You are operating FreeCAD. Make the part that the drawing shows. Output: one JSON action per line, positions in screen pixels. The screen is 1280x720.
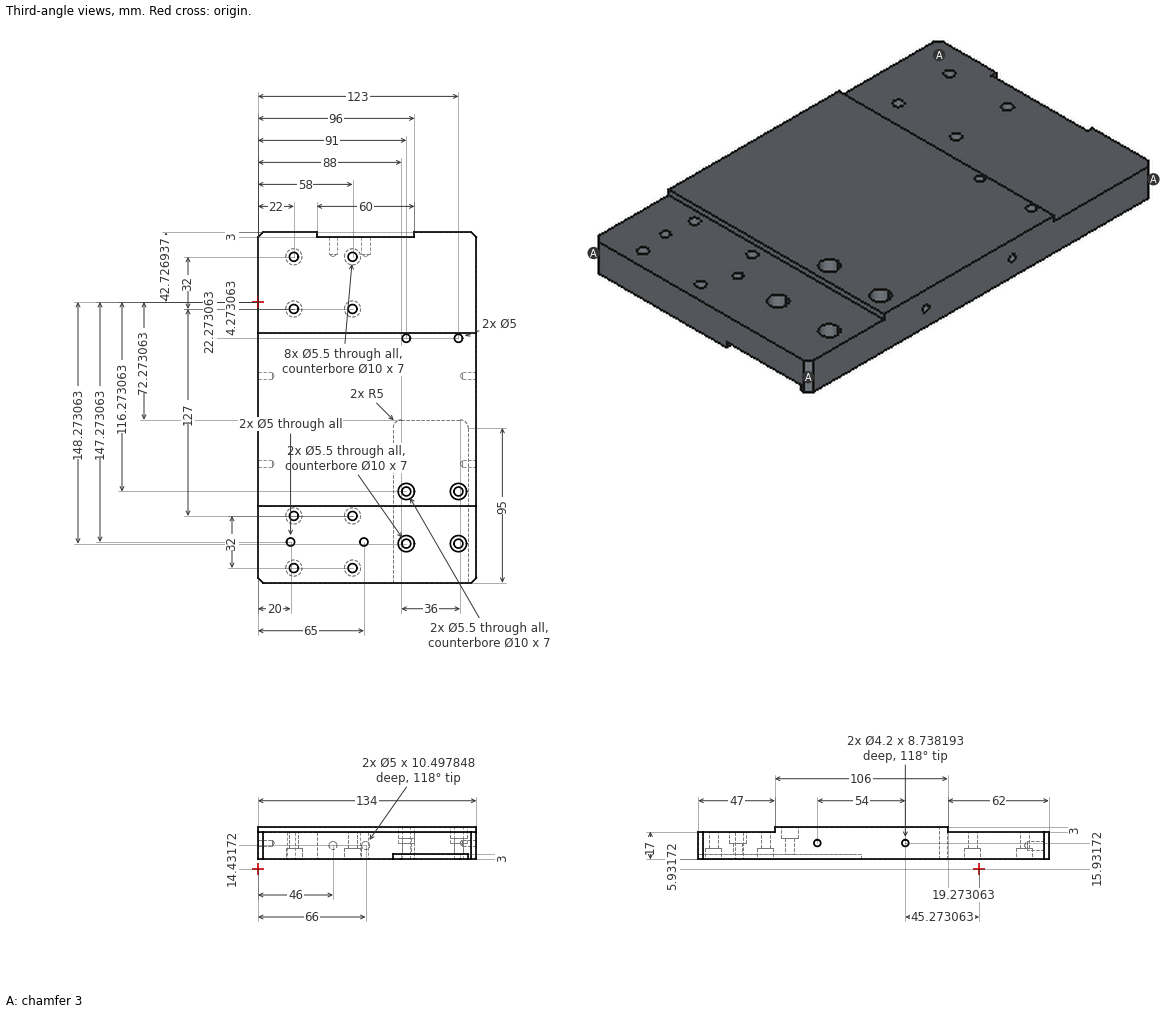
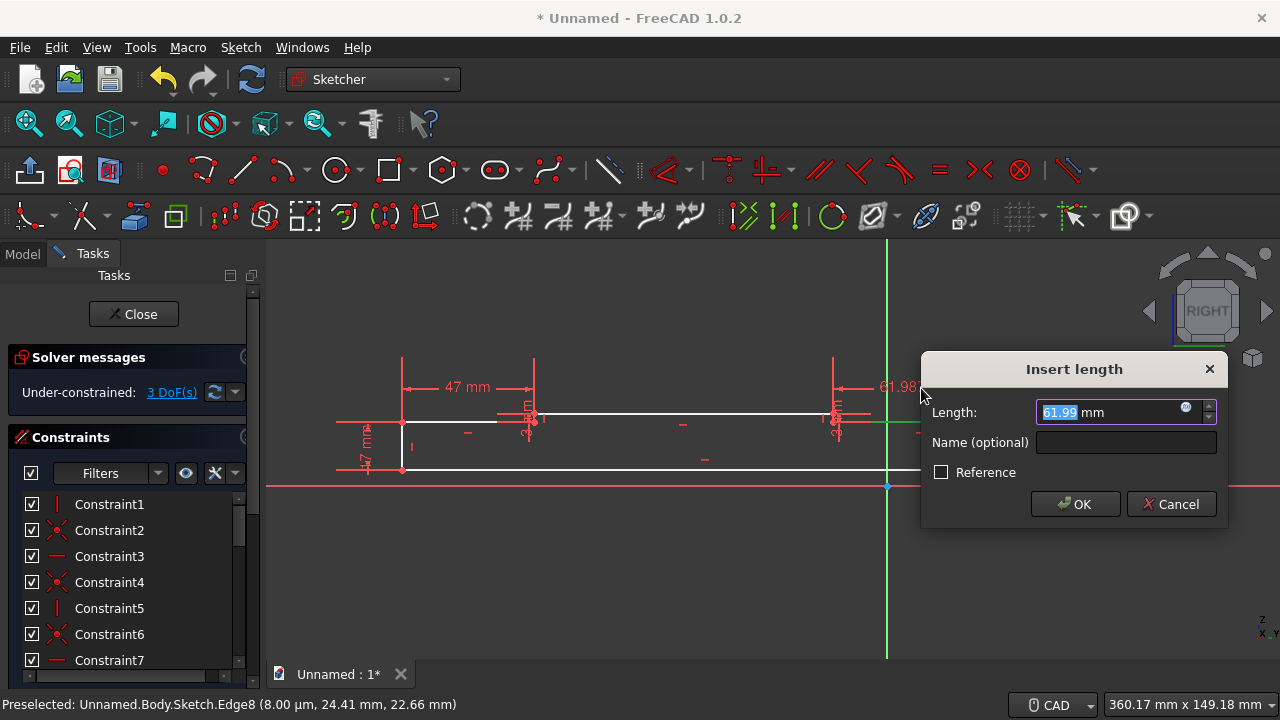
{"action": "type", "text": "62"}
{"action": "key", "text": "Return"}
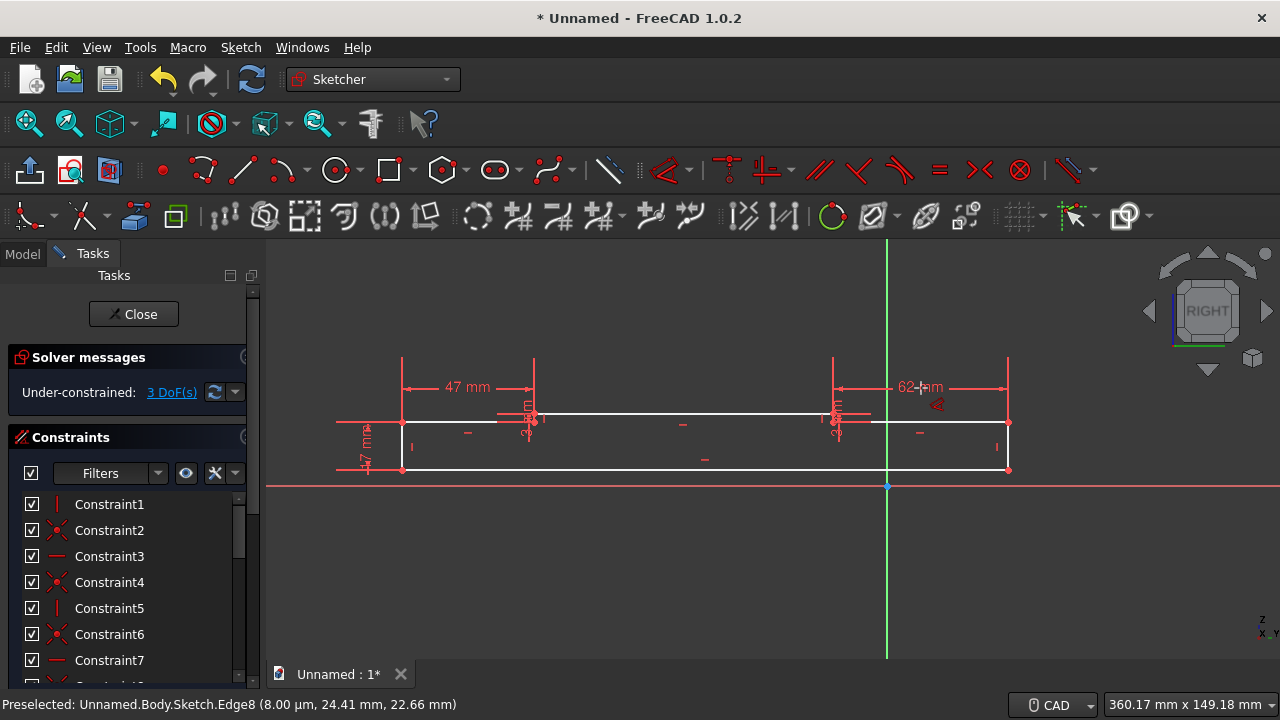
{"action": "left_click", "coordinate": [744, 414]}
{"action": "left_click", "coordinate": [684, 380]}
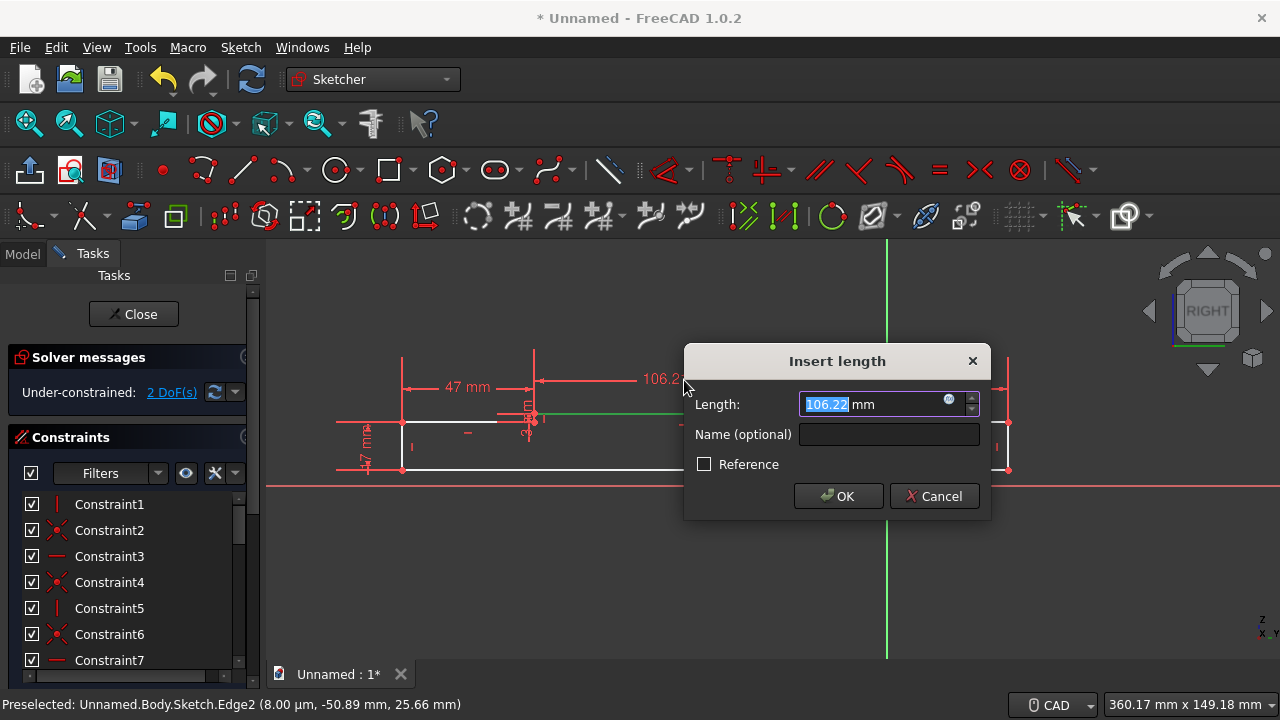
{"action": "type", "text": "106"}
{"action": "key", "text": "Return"}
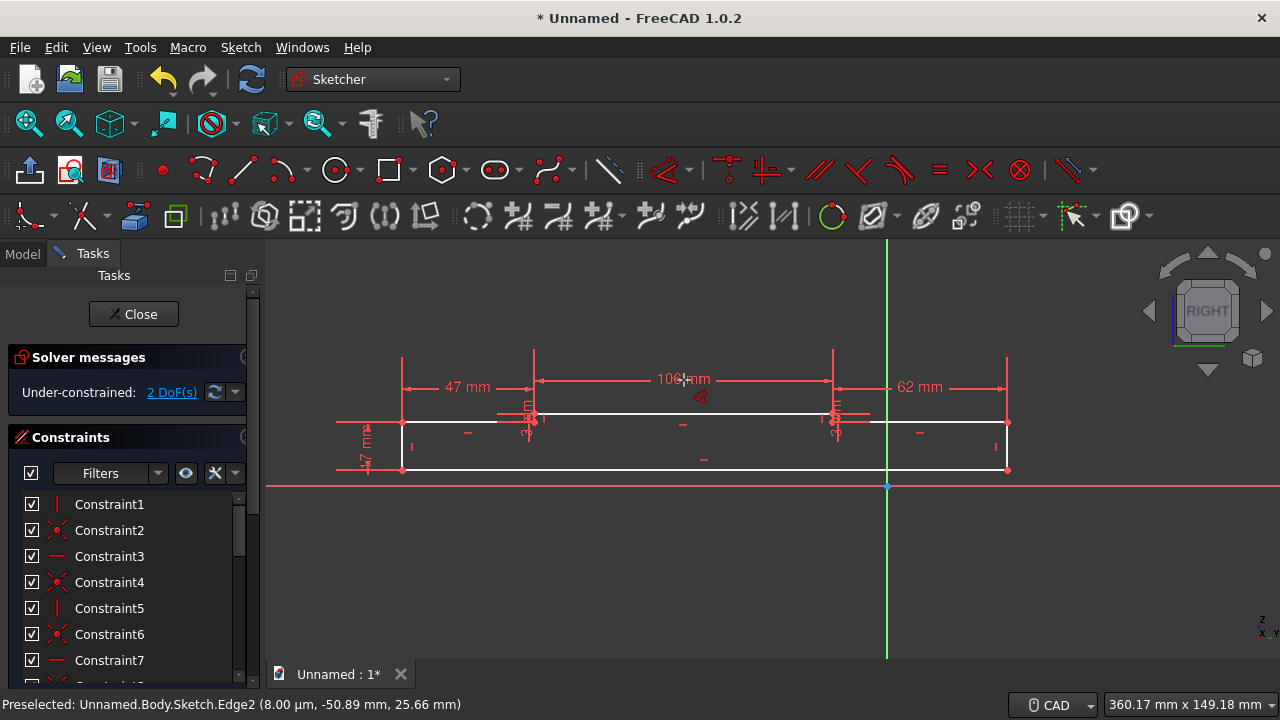
{"action": "scroll", "coordinate": [402, 470], "scroll_direction": "up", "scroll_amount": 5}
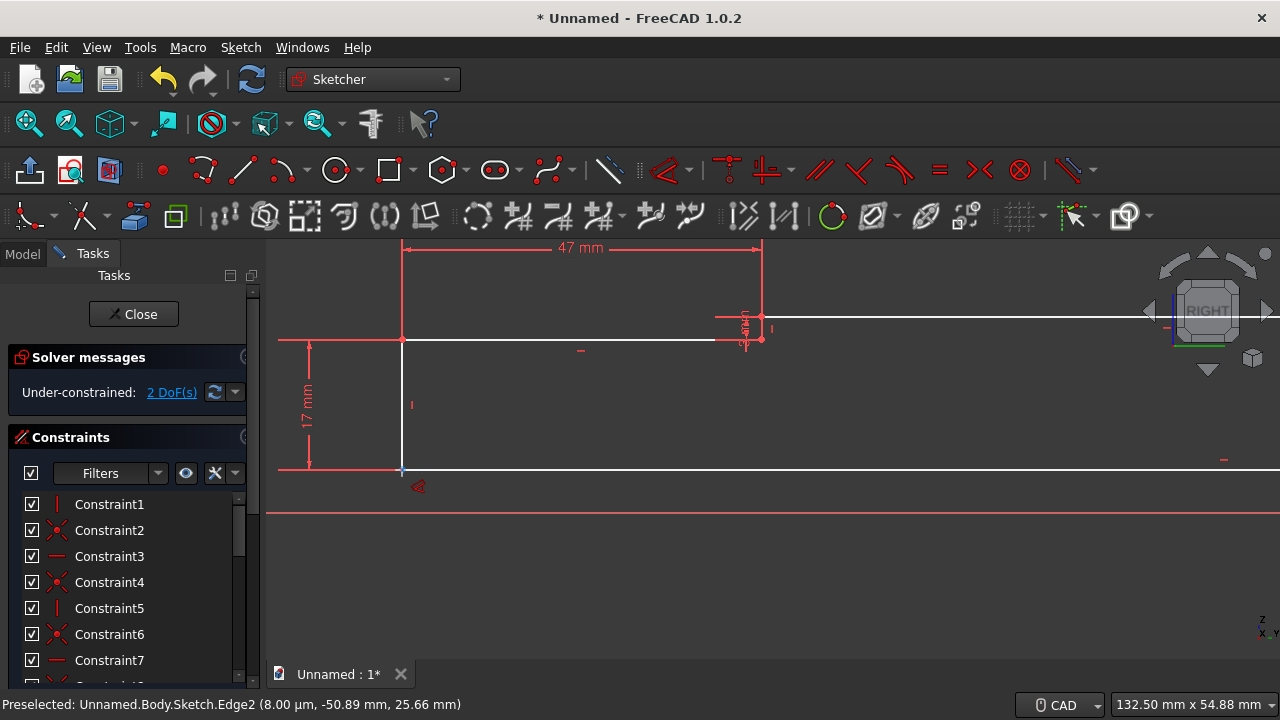
{"action": "left_click", "coordinate": [402, 470]}
{"action": "left_click", "coordinate": [368, 491]}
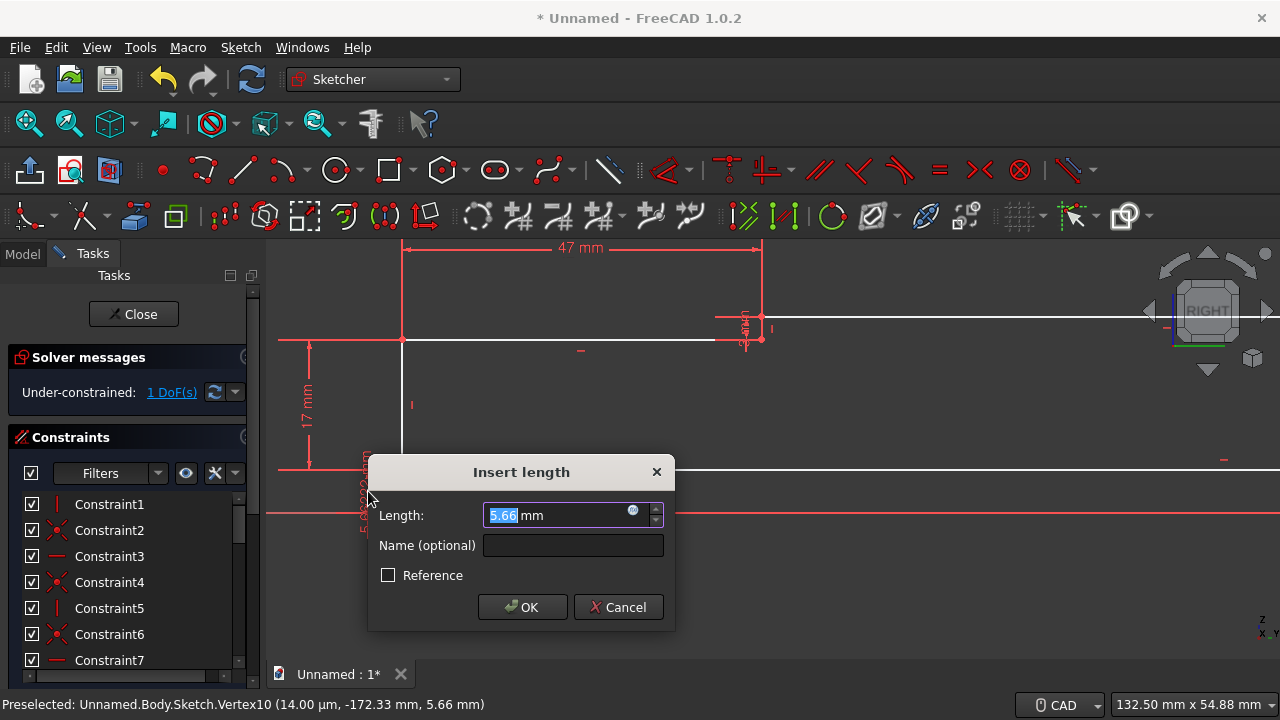
{"action": "type", "text": "5.93172"}
{"action": "key", "text": "Return"}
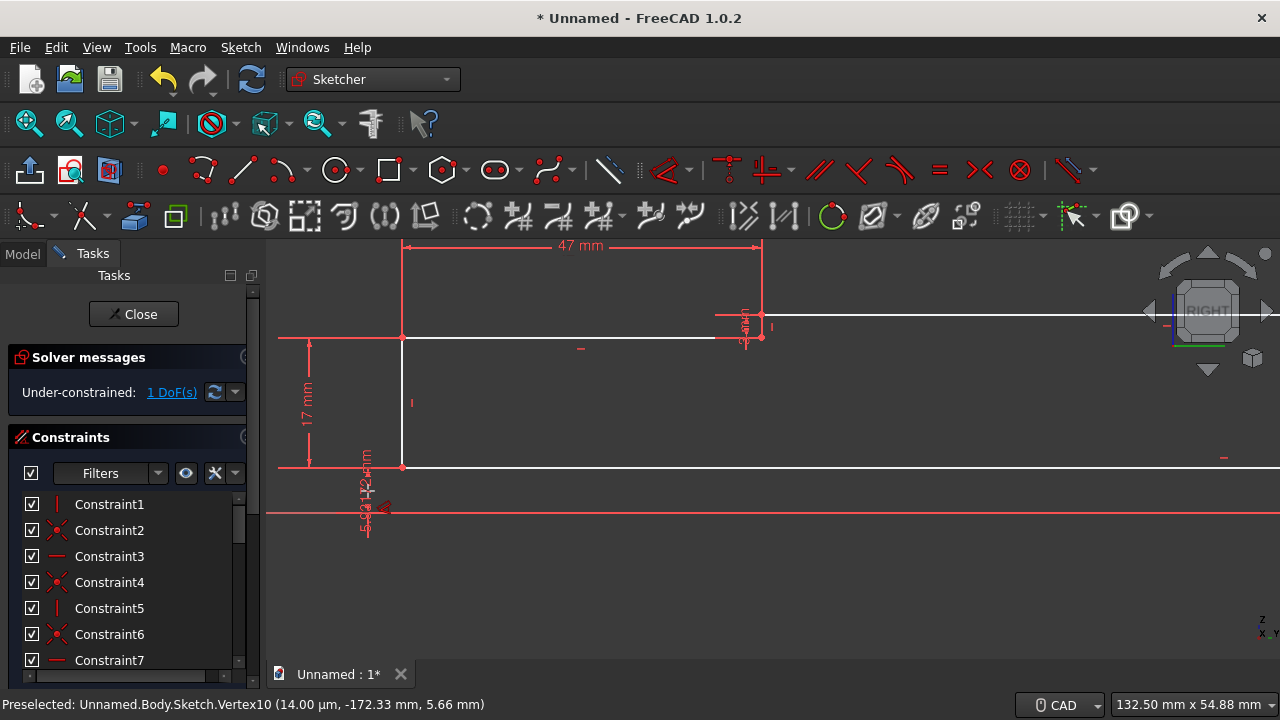
{"action": "scroll", "coordinate": [401, 469], "scroll_direction": "down", "scroll_amount": 5}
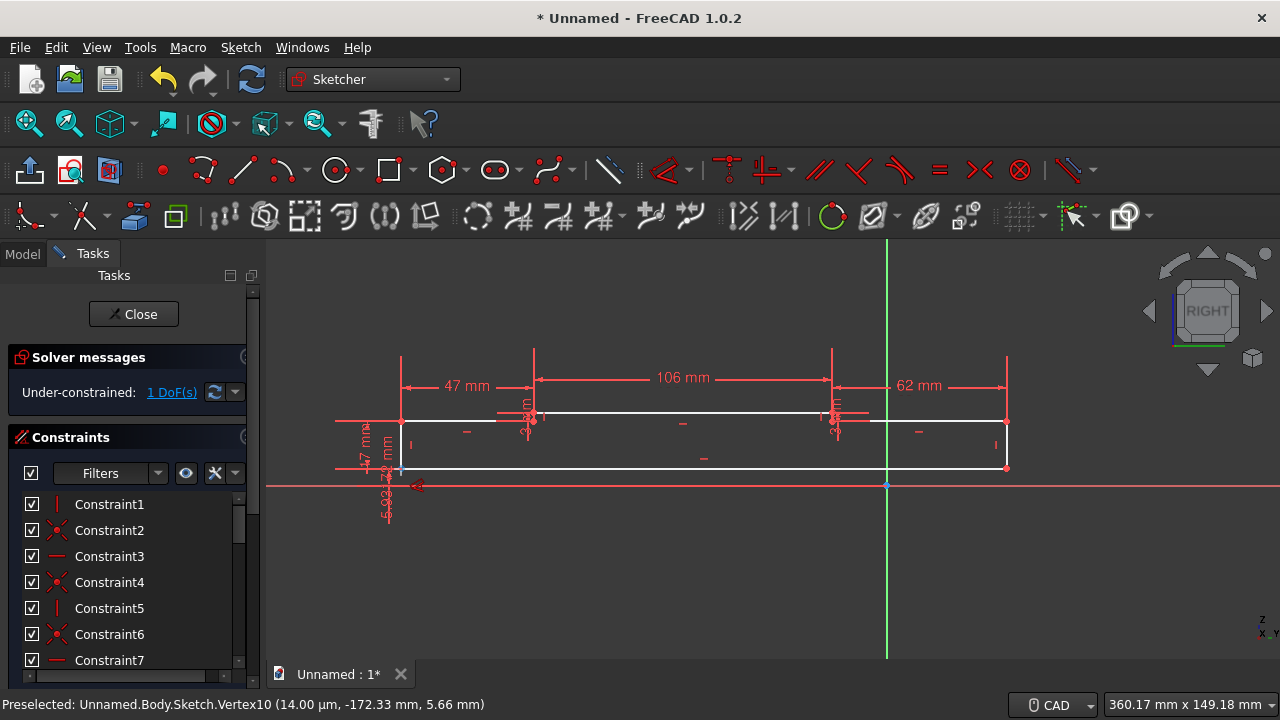
{"action": "scroll", "coordinate": [832, 421], "scroll_direction": "up", "scroll_amount": 2}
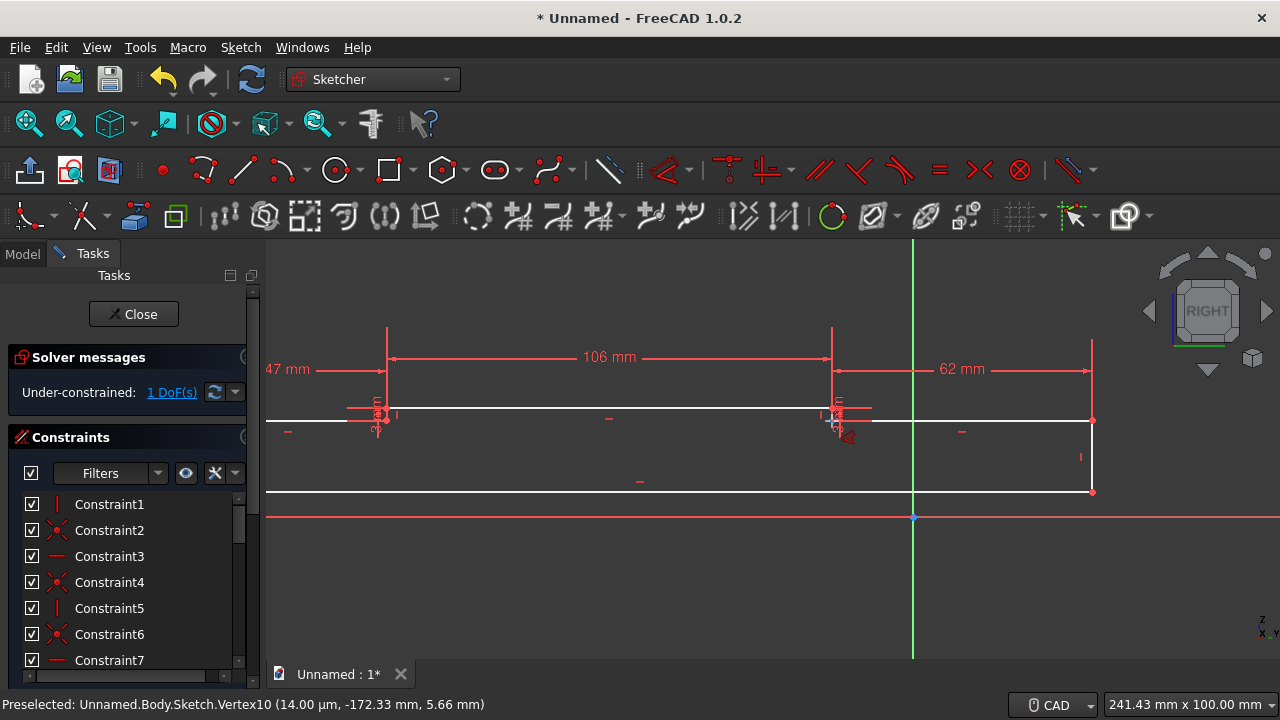
{"action": "left_click", "coordinate": [832, 421]}
{"action": "left_click", "coordinate": [873, 551]}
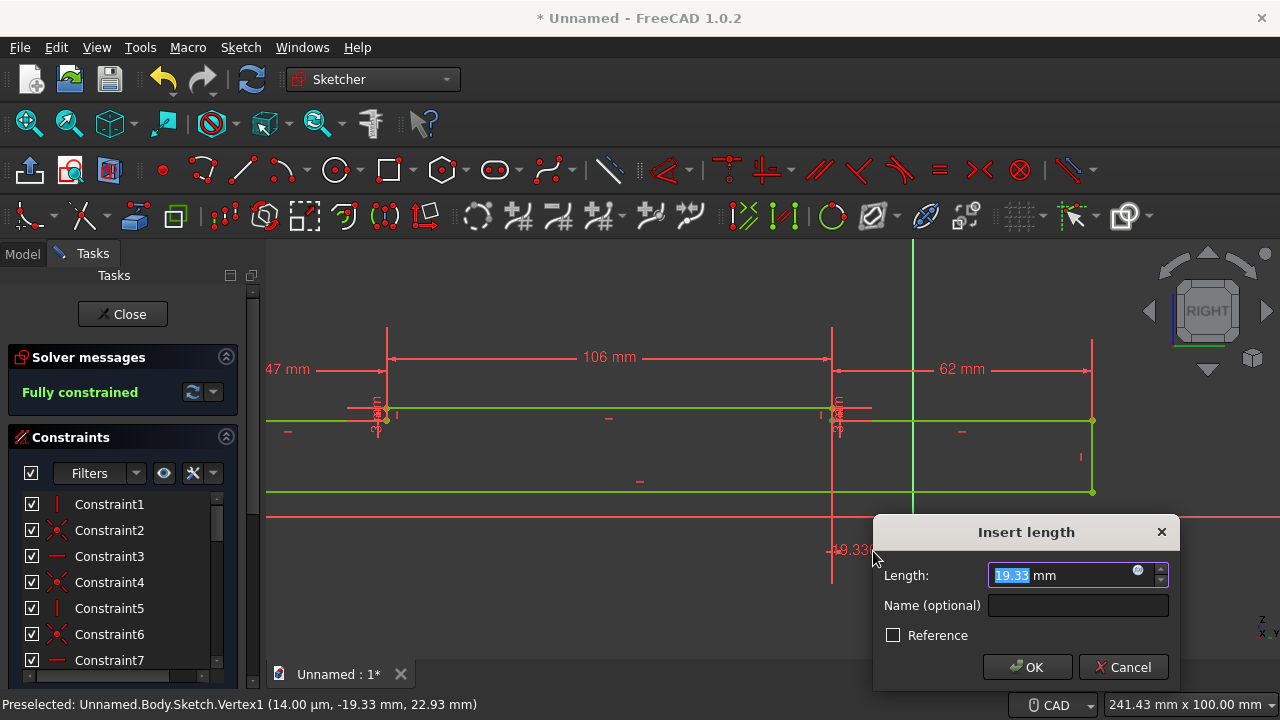
{"action": "type", "text": "19.273063"}
{"action": "key", "text": "Return"}
{"action": "key", "text": "Escape"}